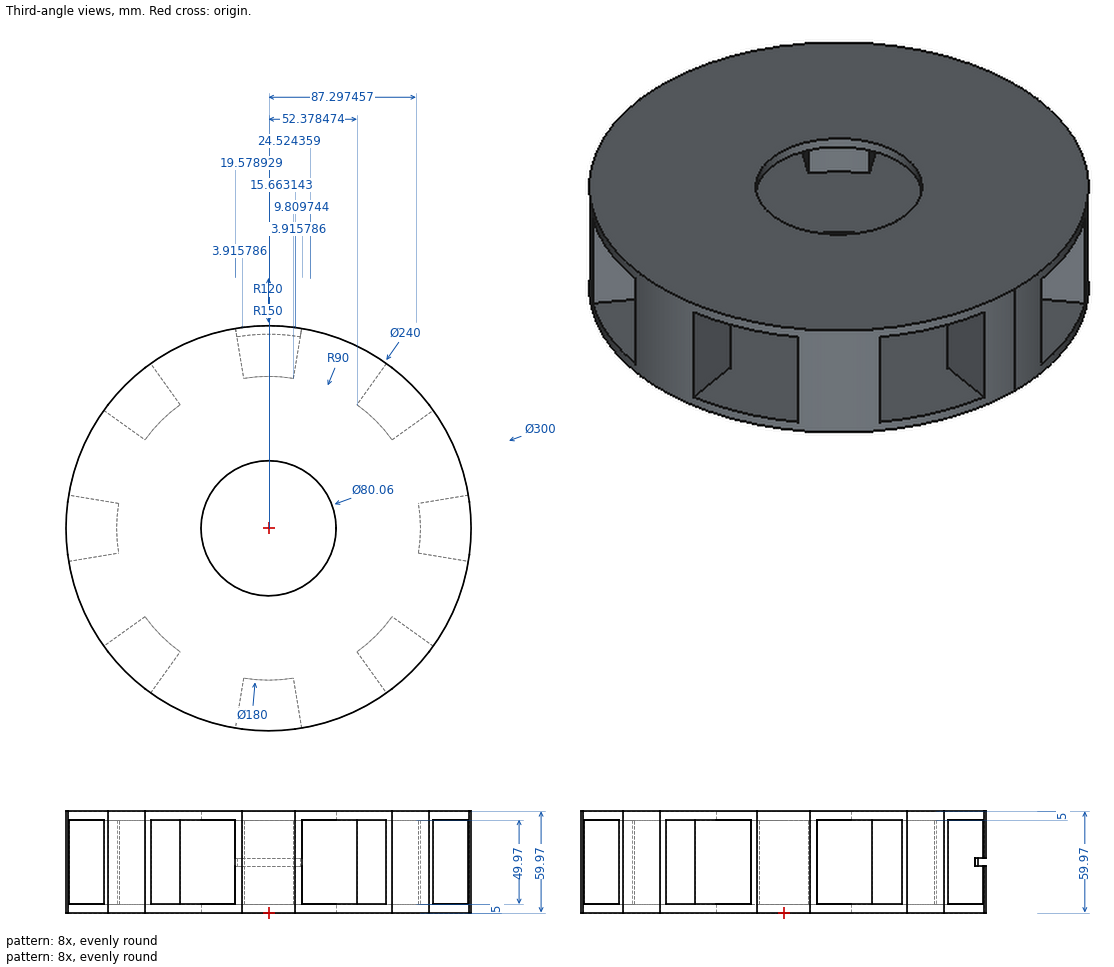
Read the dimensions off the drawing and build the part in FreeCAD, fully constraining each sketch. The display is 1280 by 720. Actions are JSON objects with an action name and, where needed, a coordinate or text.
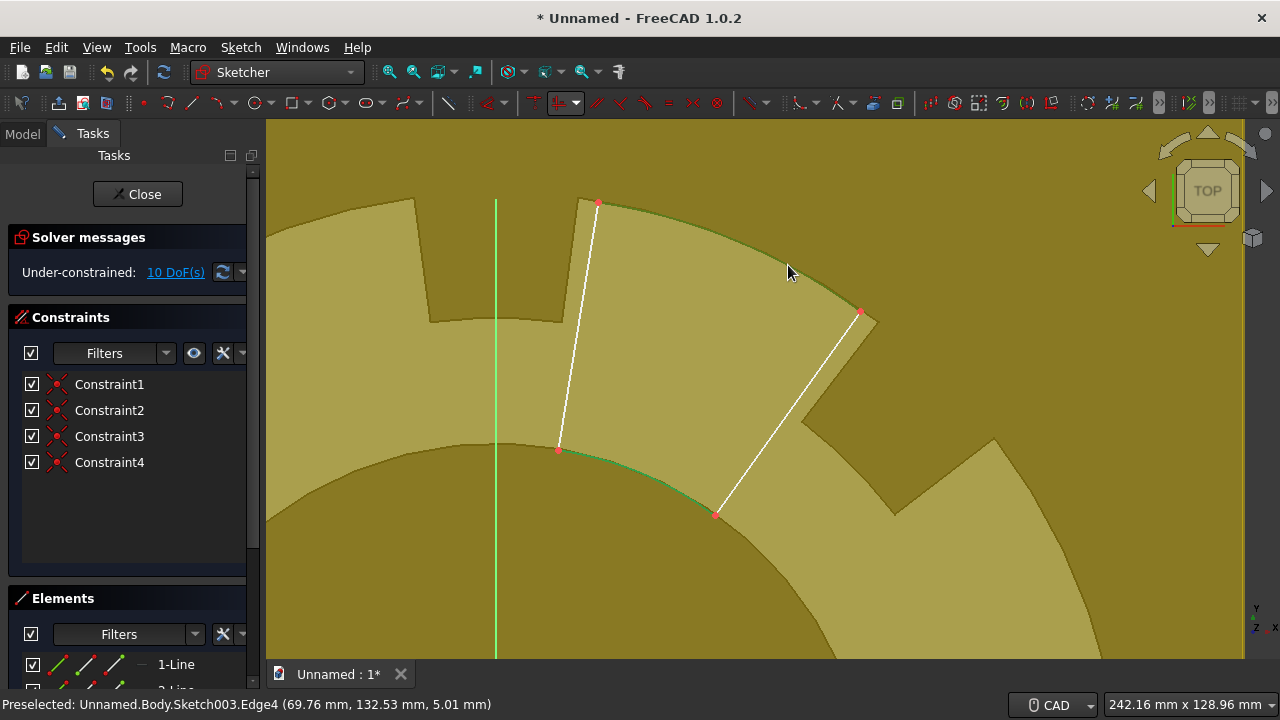
{"action": "left_click", "coordinate": [534, 104]}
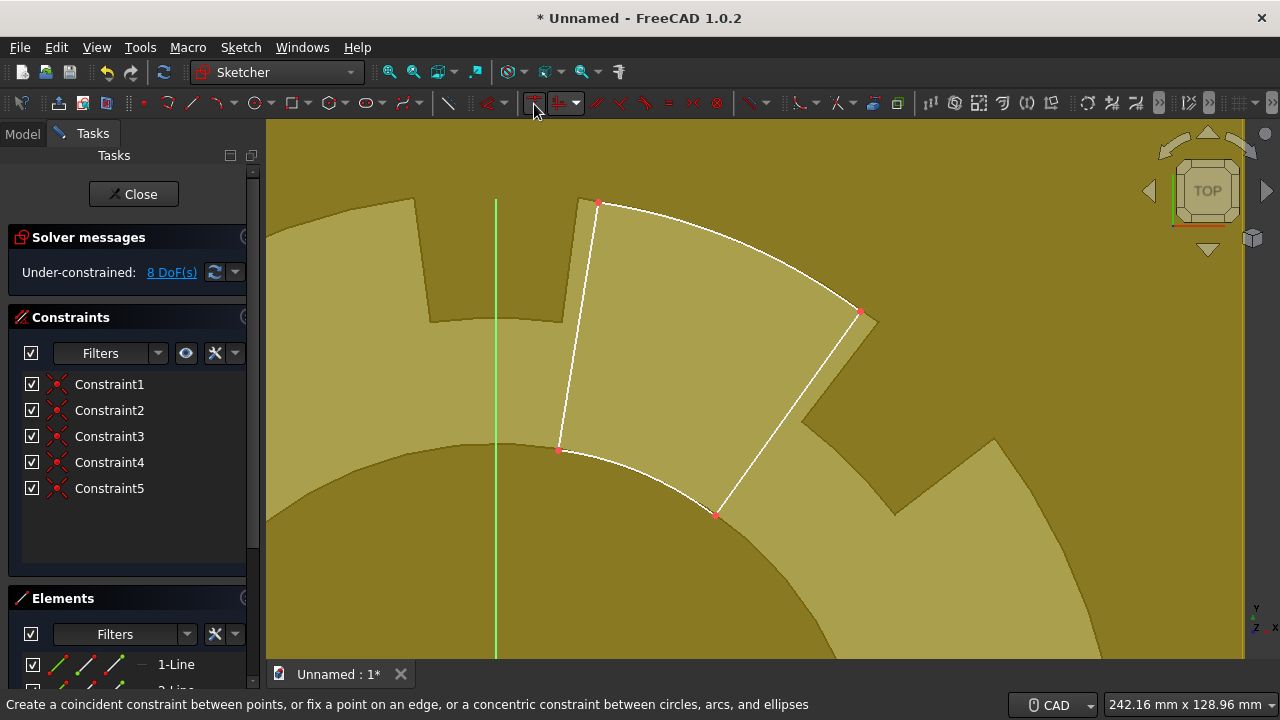
{"action": "scroll", "coordinate": [736, 241], "scroll_direction": "down", "scroll_amount": 3}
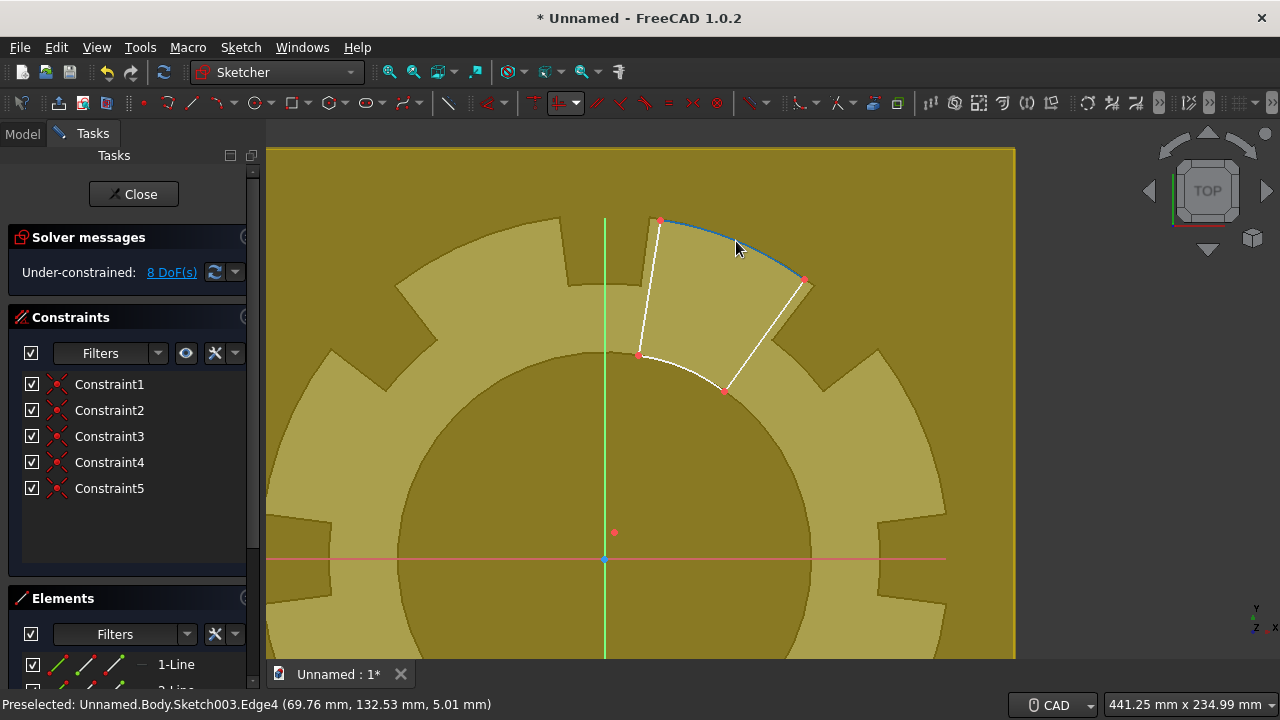
{"action": "left_click_drag", "start_coordinate": [595, 523], "coordinate": [625, 569]}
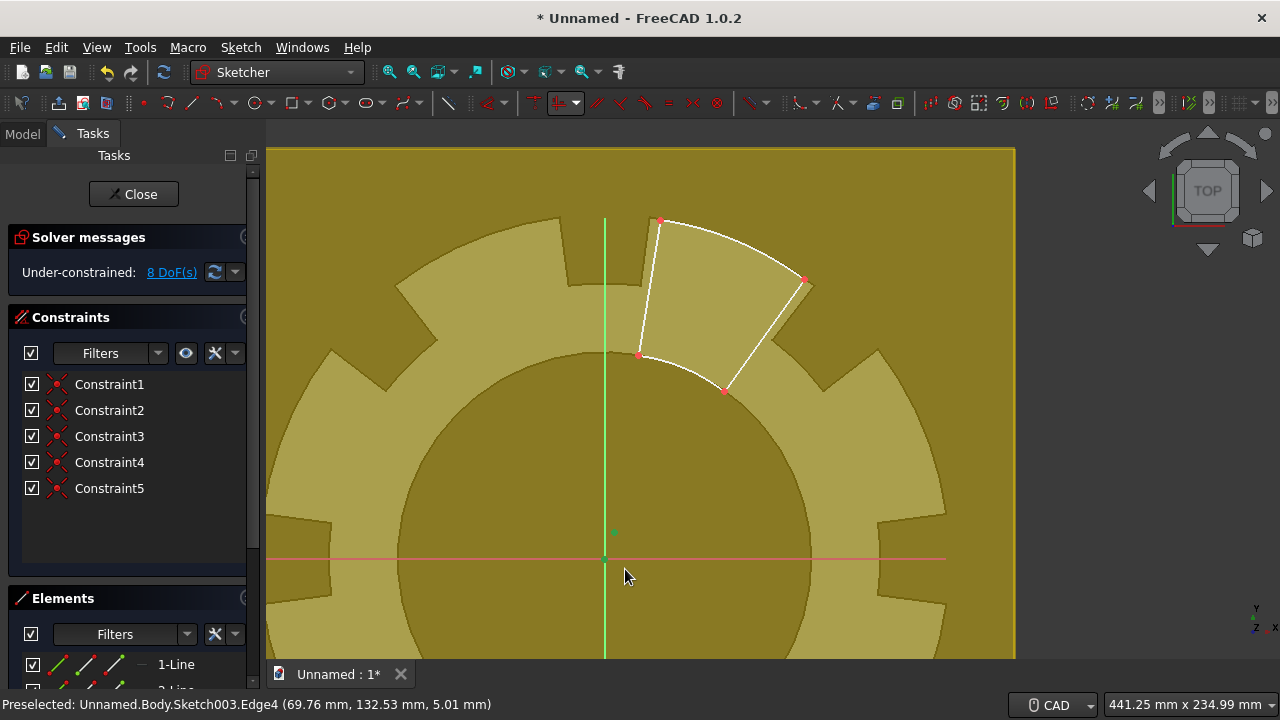
{"action": "left_click", "coordinate": [534, 104]}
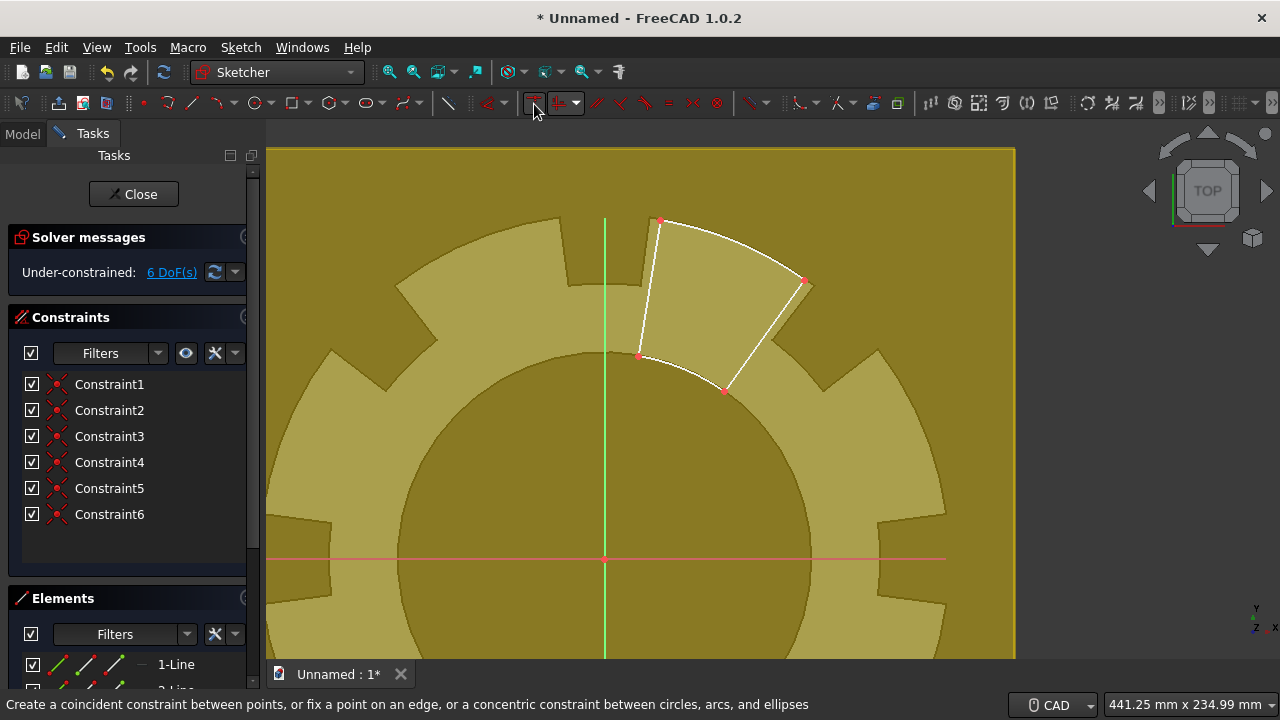
{"action": "left_click", "coordinate": [488, 104]}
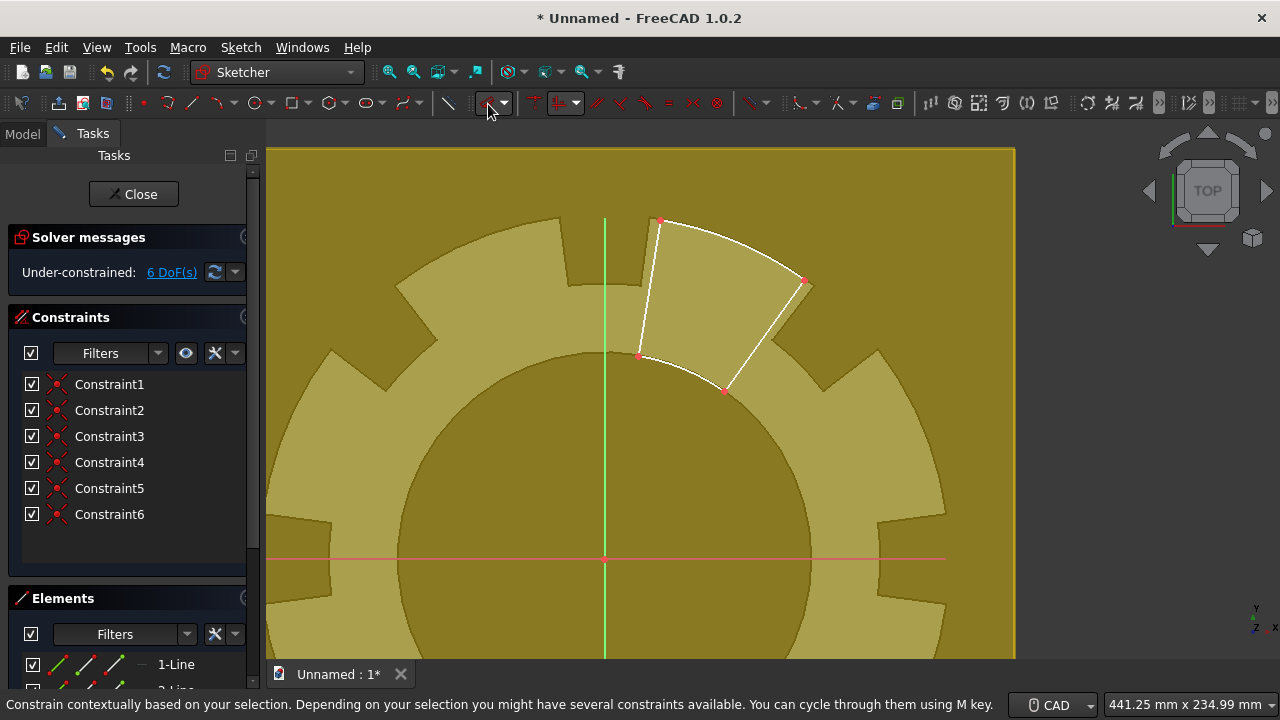
{"action": "left_click", "coordinate": [701, 377]}
{"action": "left_click", "coordinate": [716, 349]}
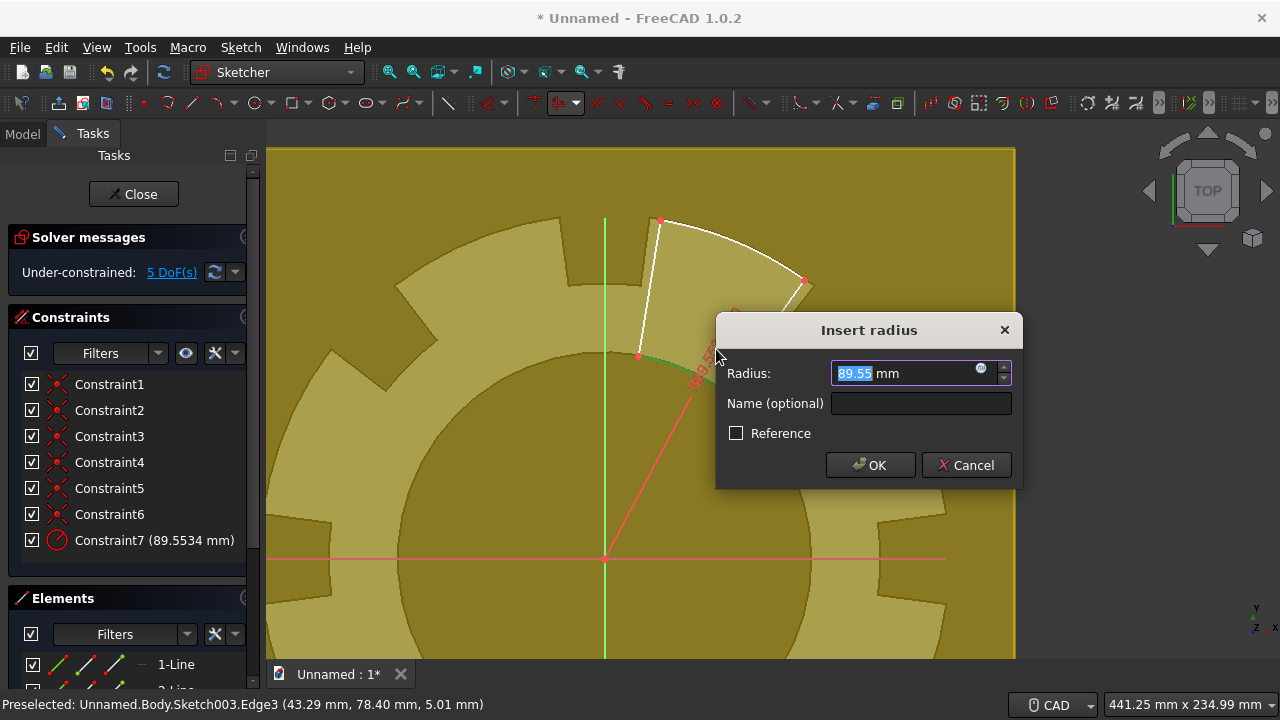
{"action": "type", "text": "90"}
{"action": "key", "text": "Return"}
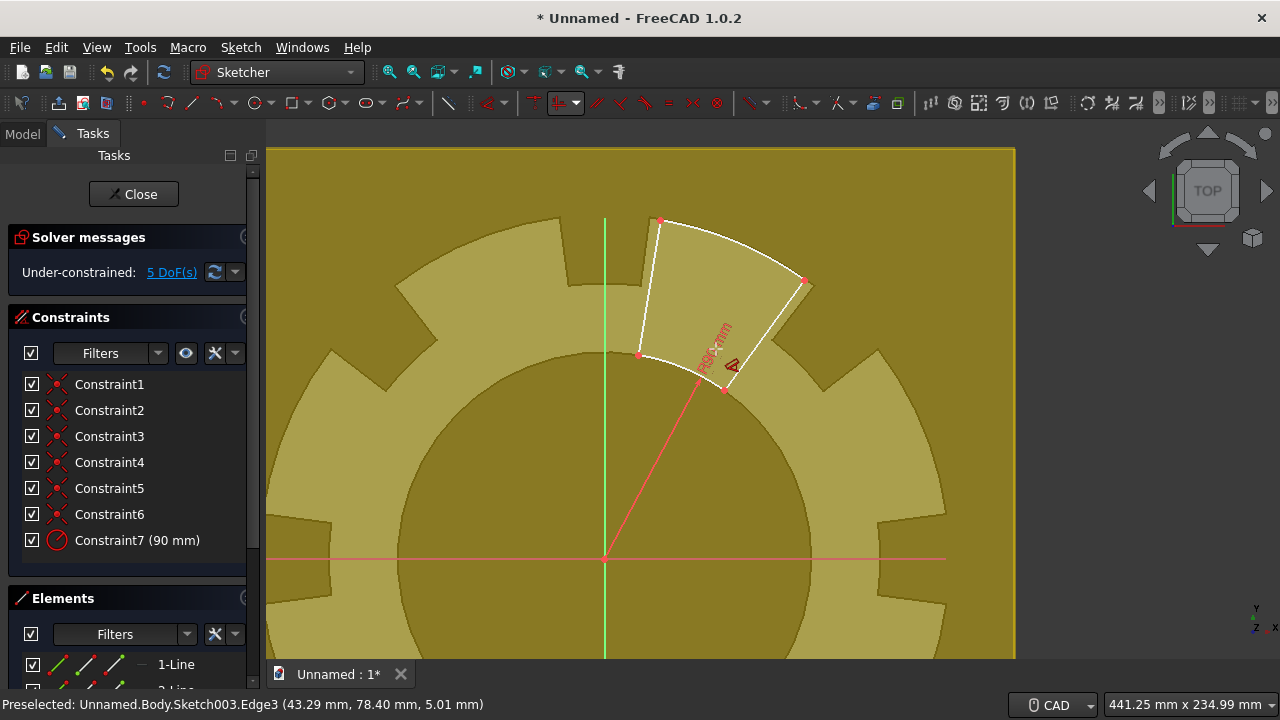
{"action": "left_click", "coordinate": [765, 255]}
{"action": "left_click", "coordinate": [780, 227]}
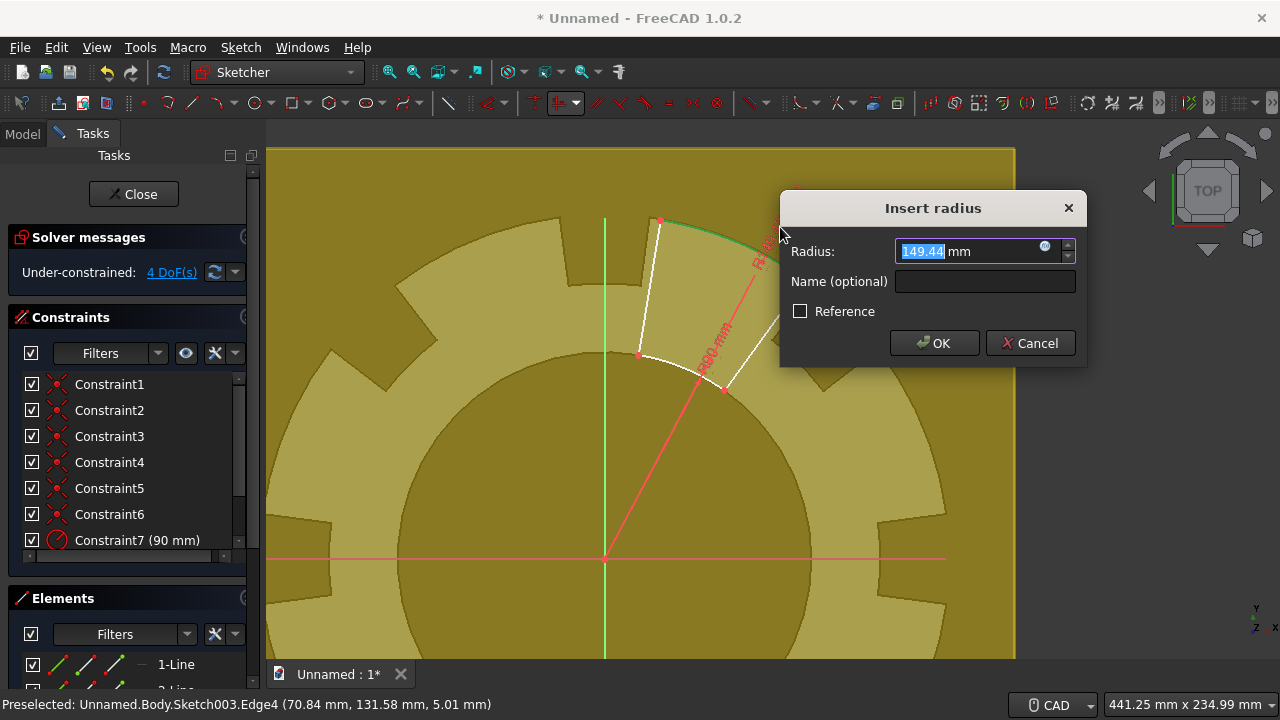
{"action": "type", "text": "150"}
{"action": "key", "text": "Return"}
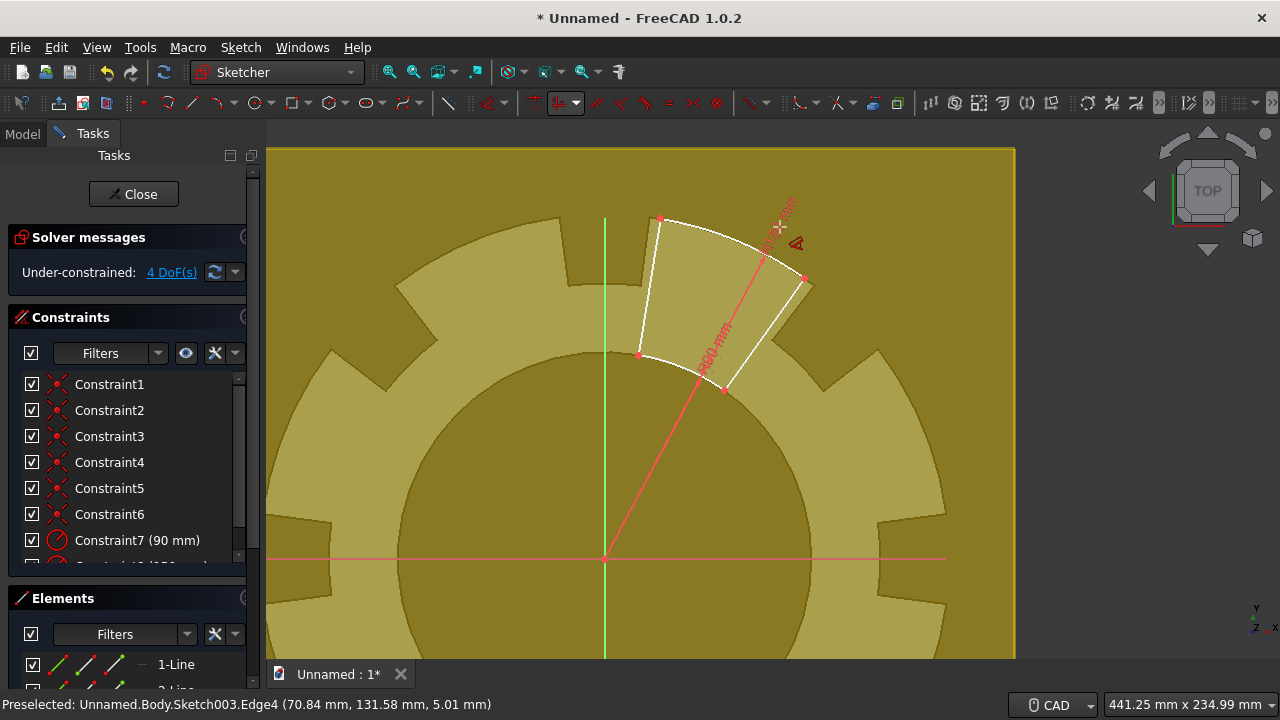
{"action": "scroll", "coordinate": [654, 260], "scroll_direction": "up", "scroll_amount": 3}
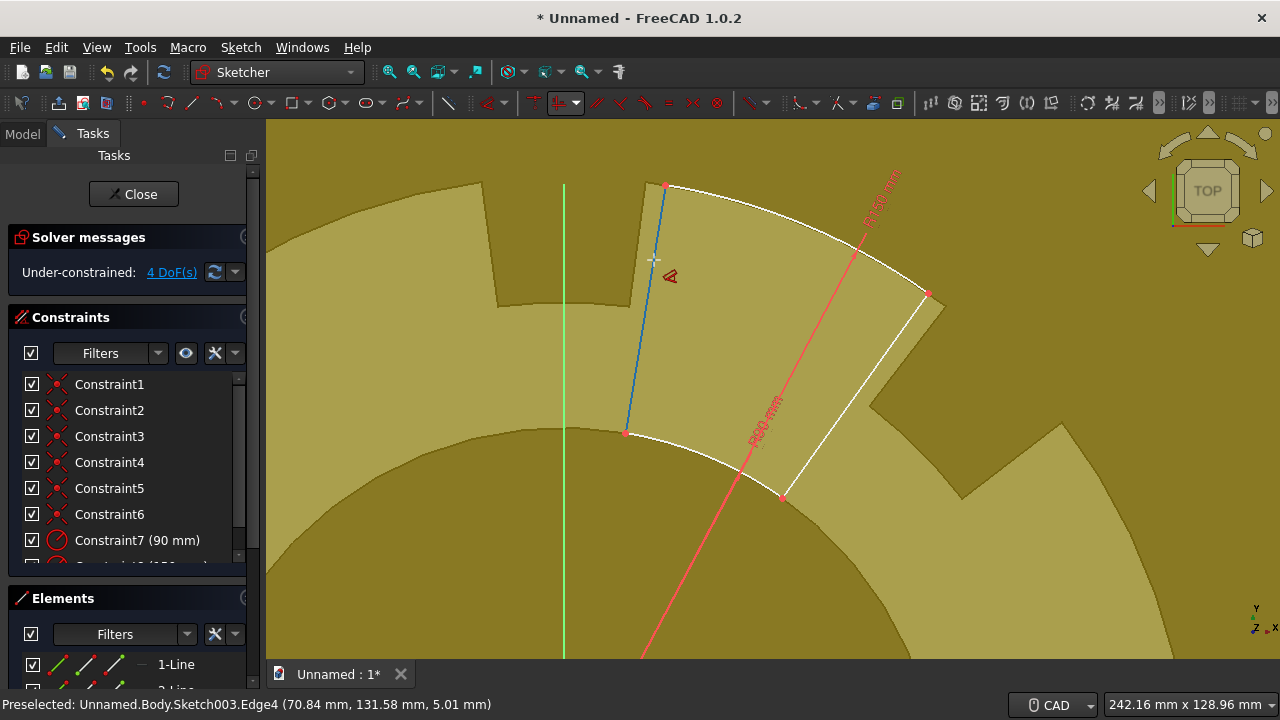
{"action": "left_click", "coordinate": [654, 259]}
{"action": "left_click", "coordinate": [646, 151]}